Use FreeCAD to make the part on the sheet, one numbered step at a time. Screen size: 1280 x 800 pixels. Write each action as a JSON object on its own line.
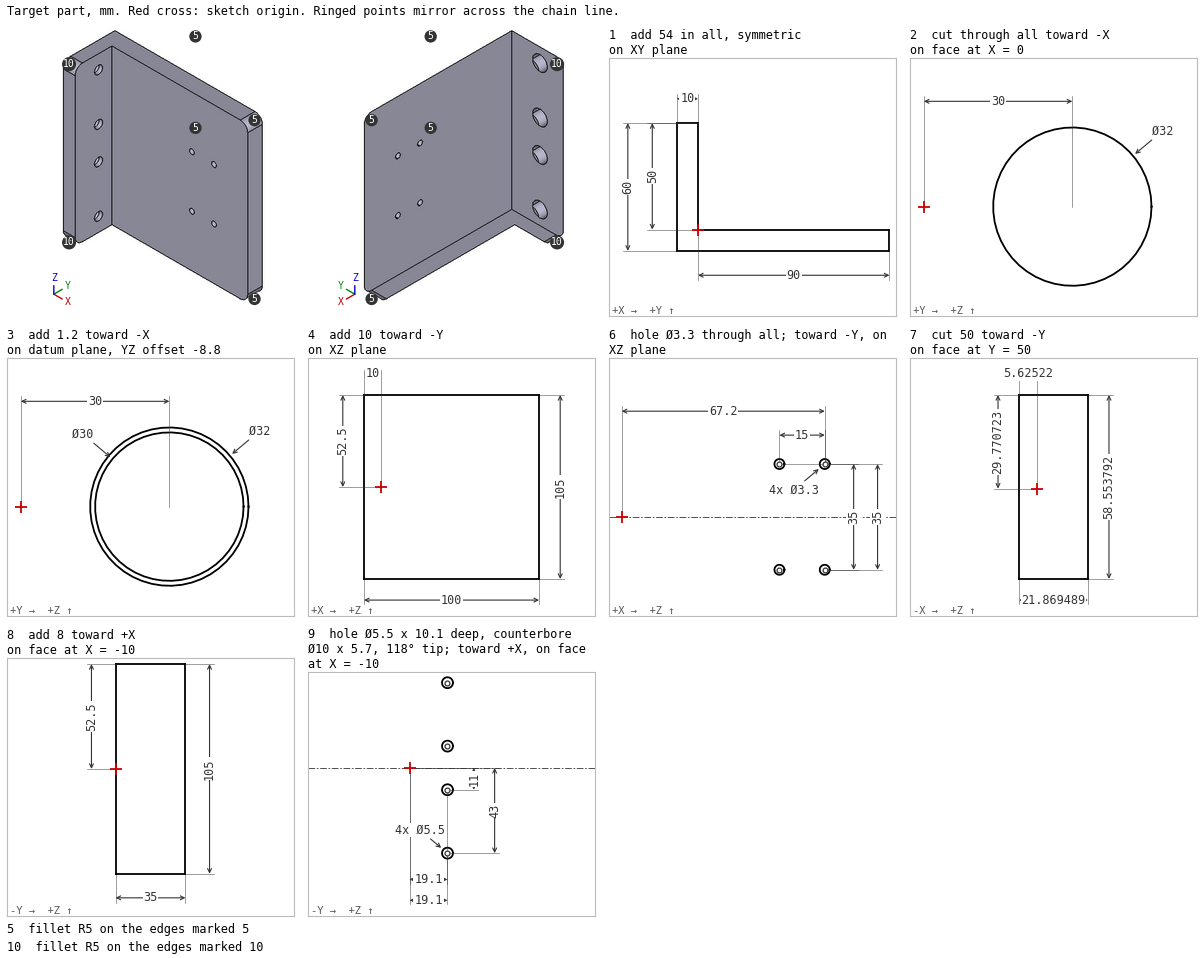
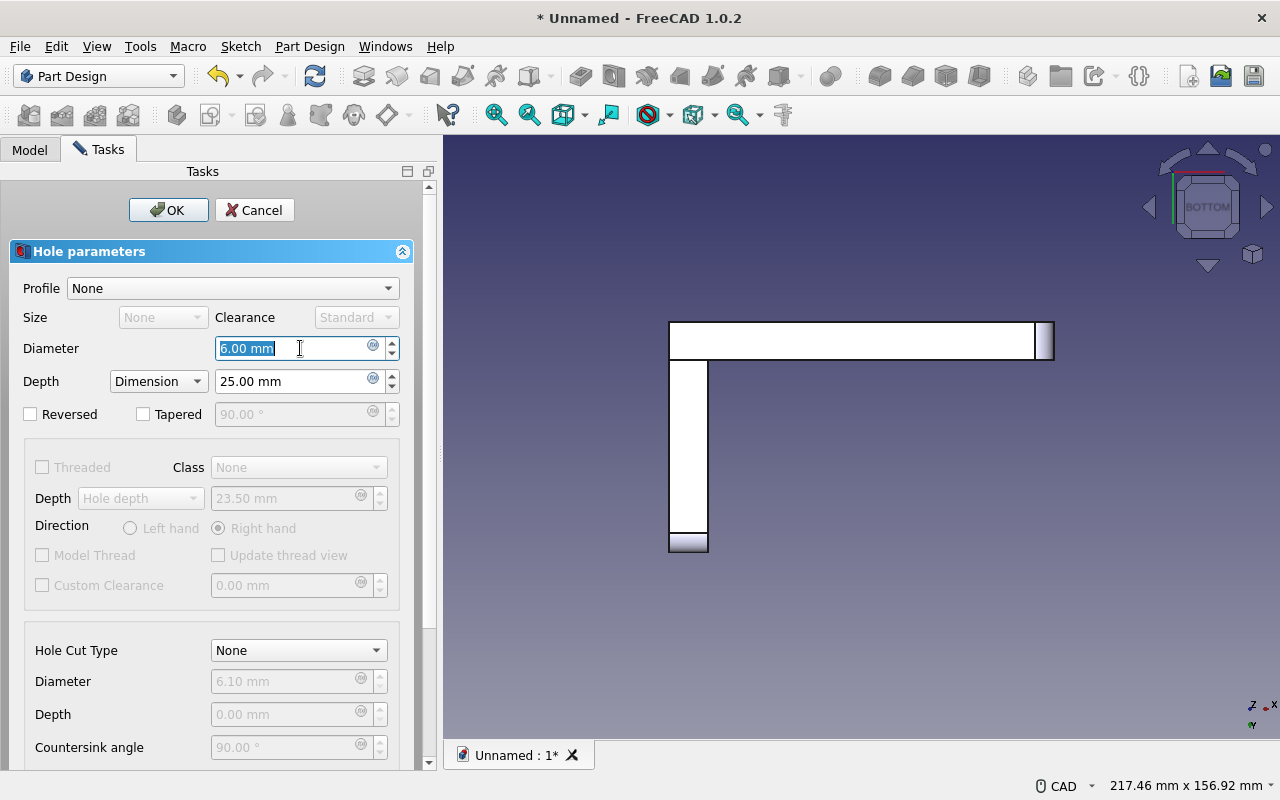
{"action": "type", "text": "3.3"}
{"action": "key", "text": "Tab"}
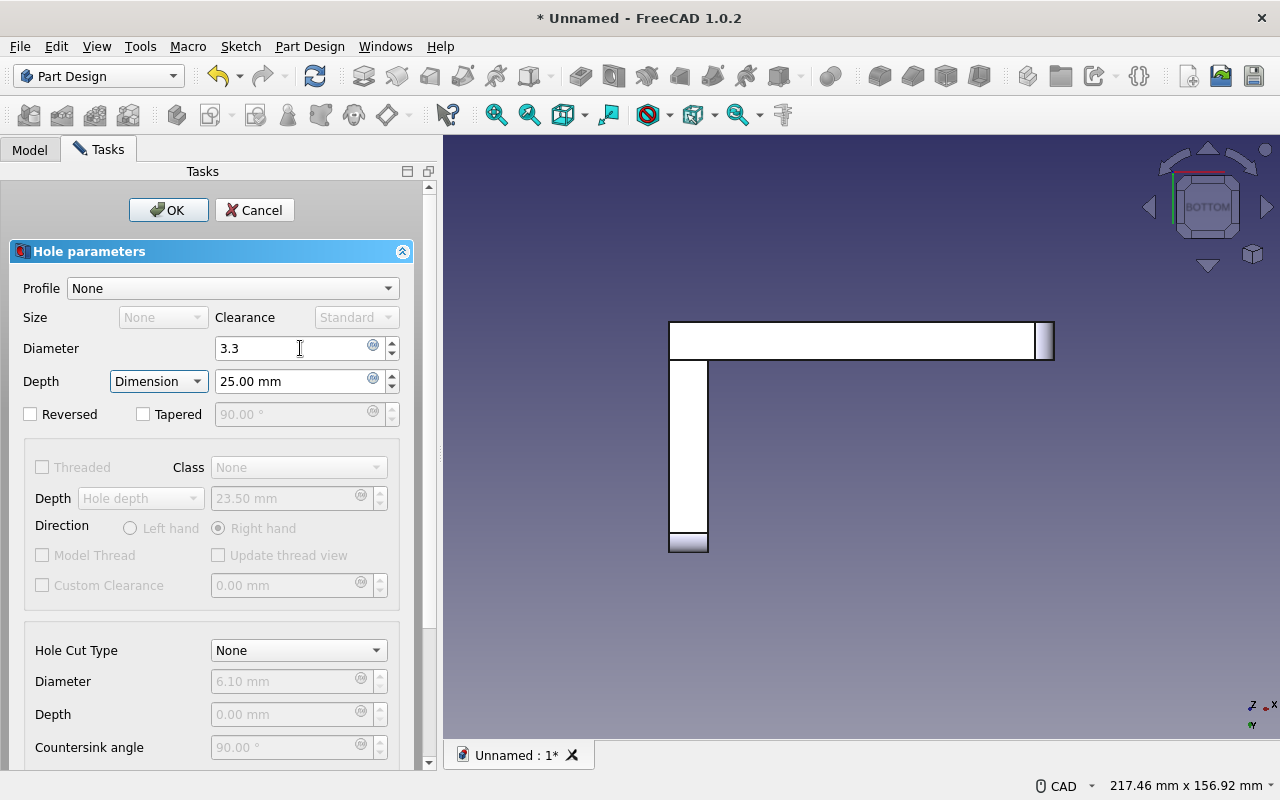
{"action": "left_click", "coordinate": [160, 382]}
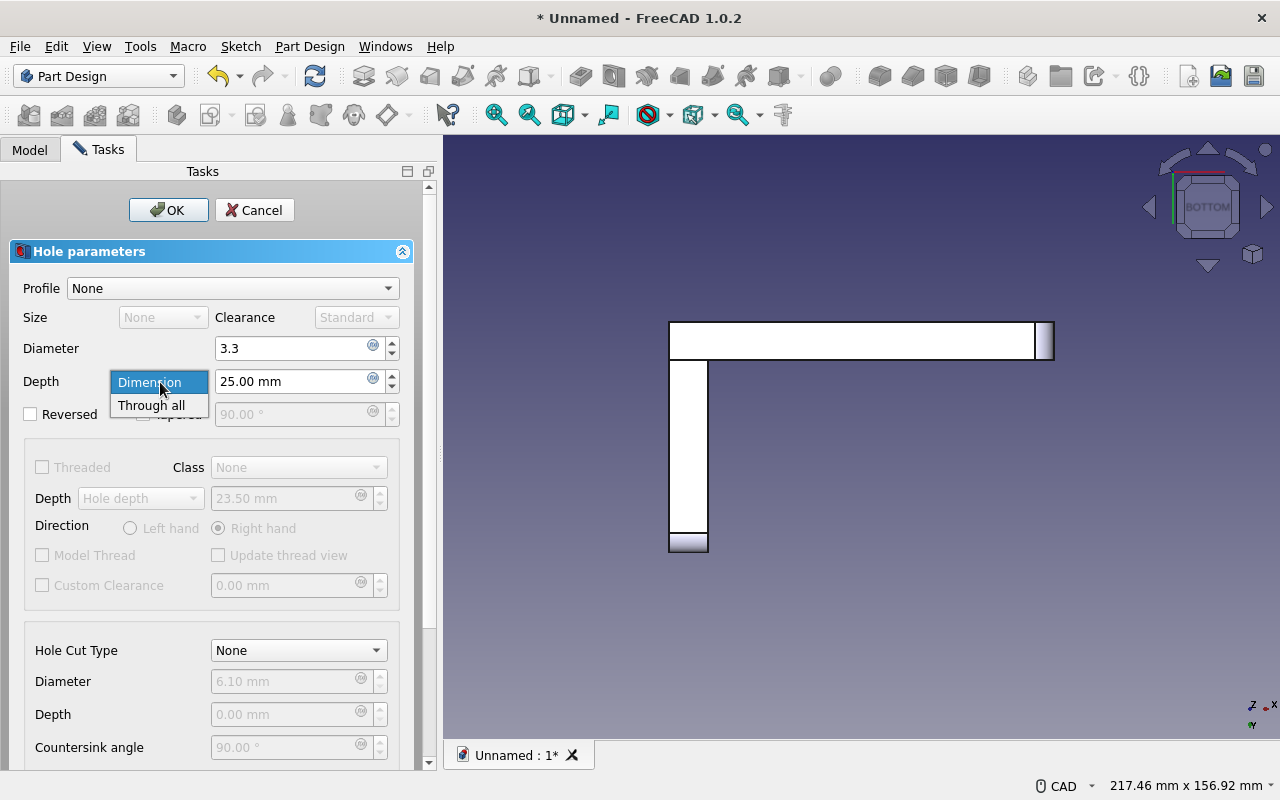
{"action": "left_click", "coordinate": [158, 406]}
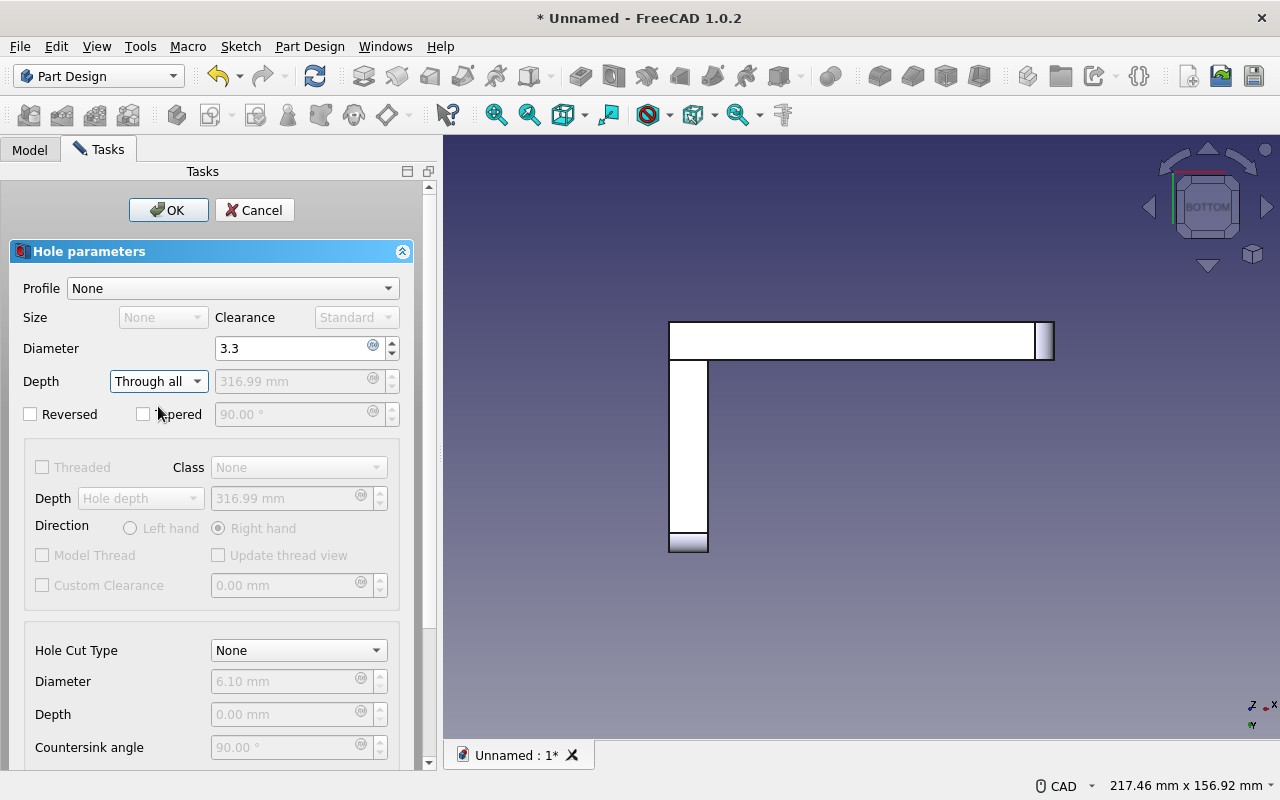
{"action": "left_click", "coordinate": [31, 414]}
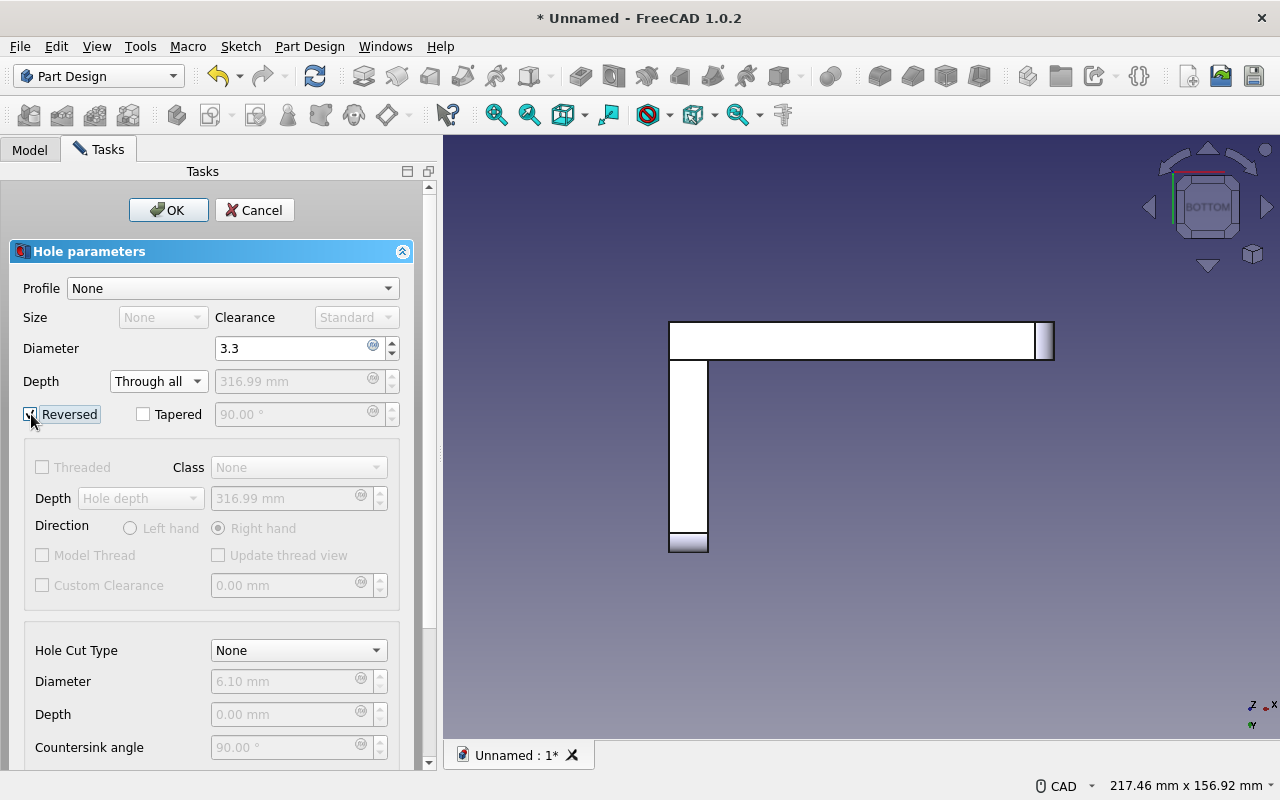
{"action": "left_click", "coordinate": [169, 210]}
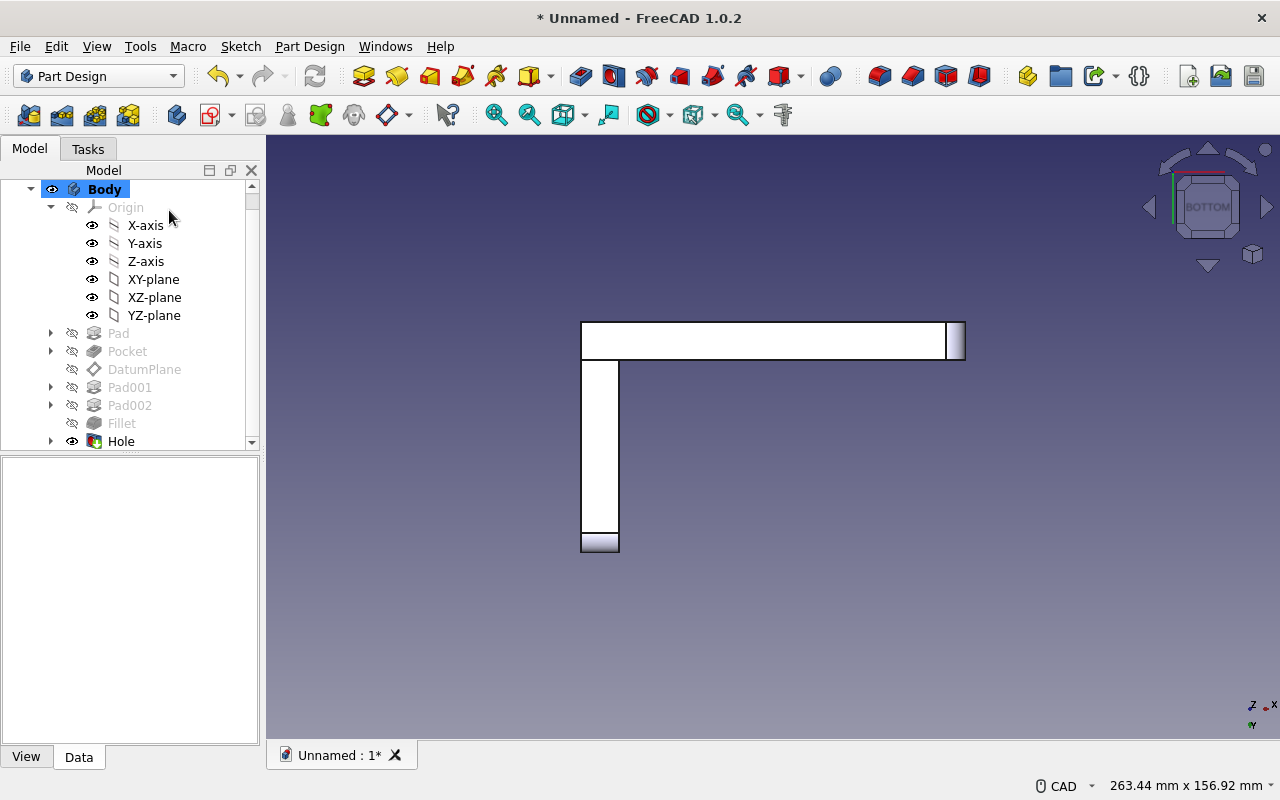
{"action": "left_click", "coordinate": [497, 116]}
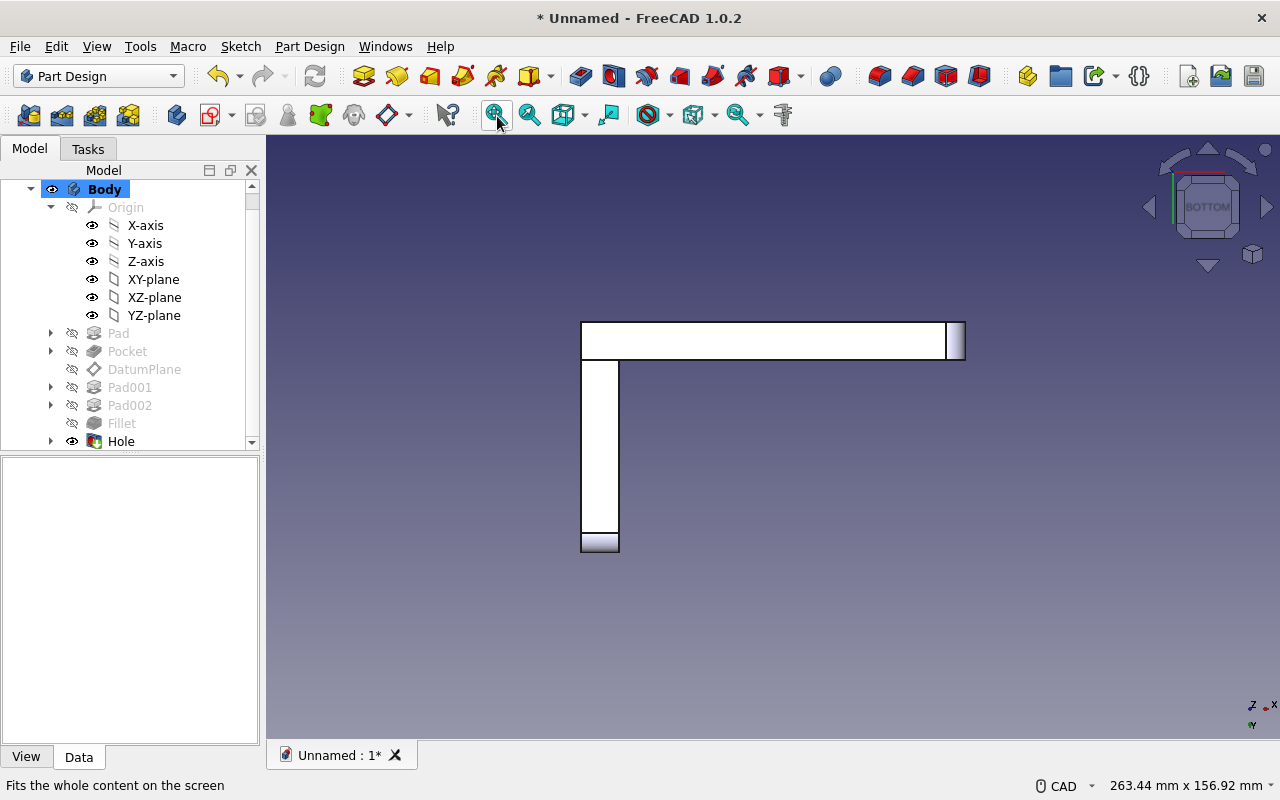
{"action": "key", "text": "4"}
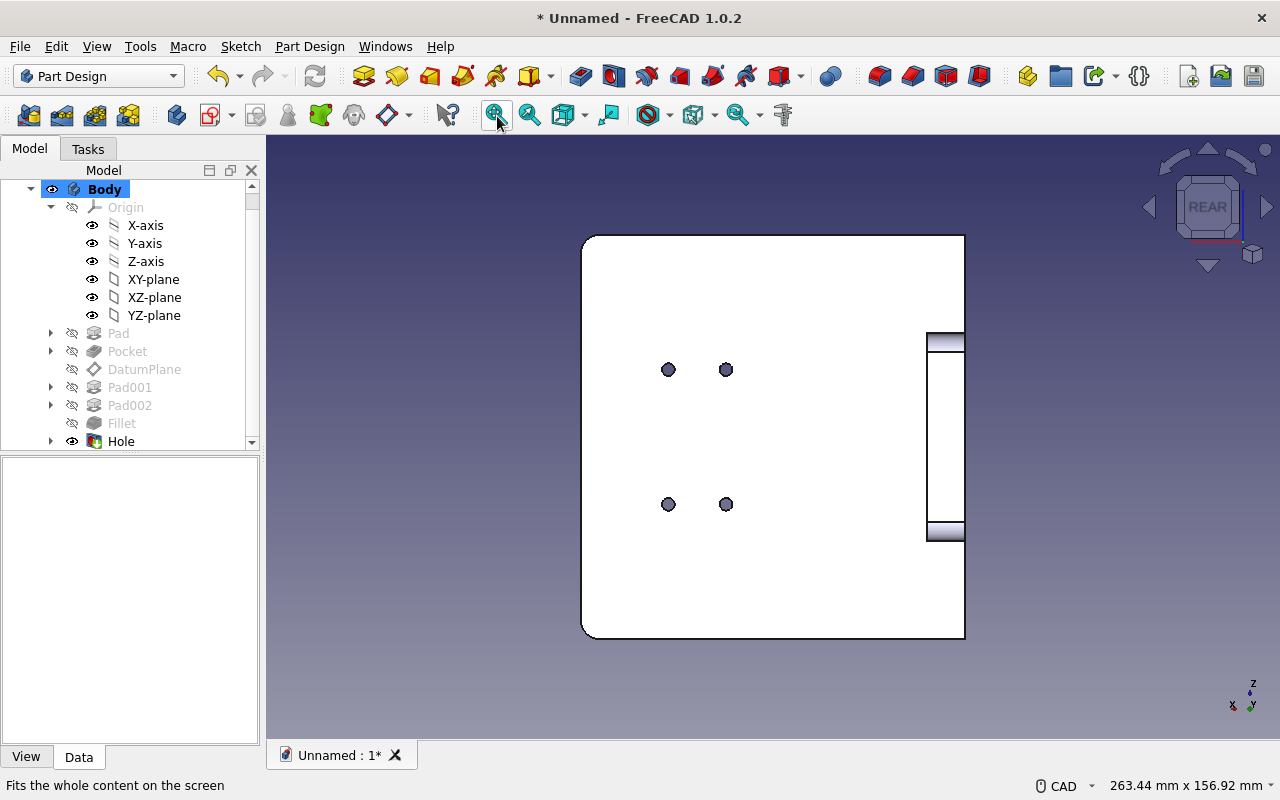
{"action": "left_click", "coordinate": [946, 388]}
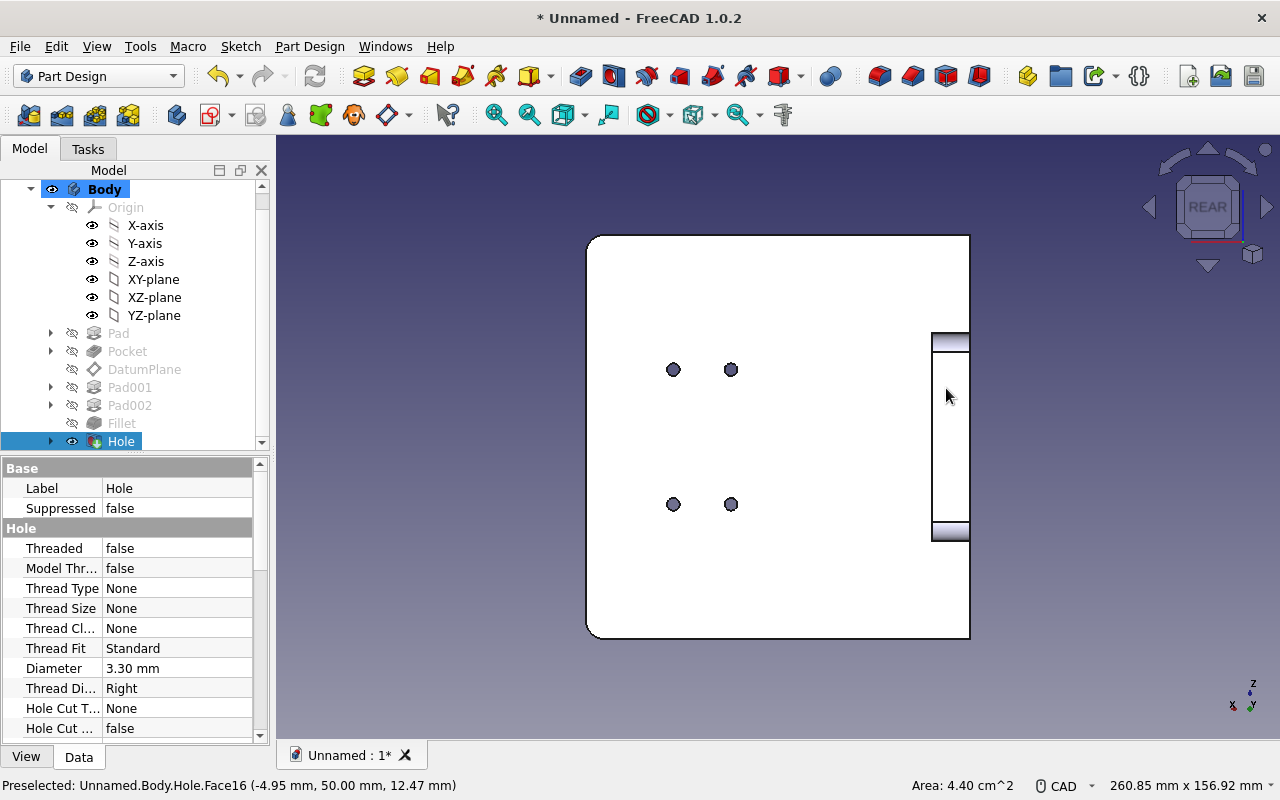
{"action": "left_click", "coordinate": [210, 116]}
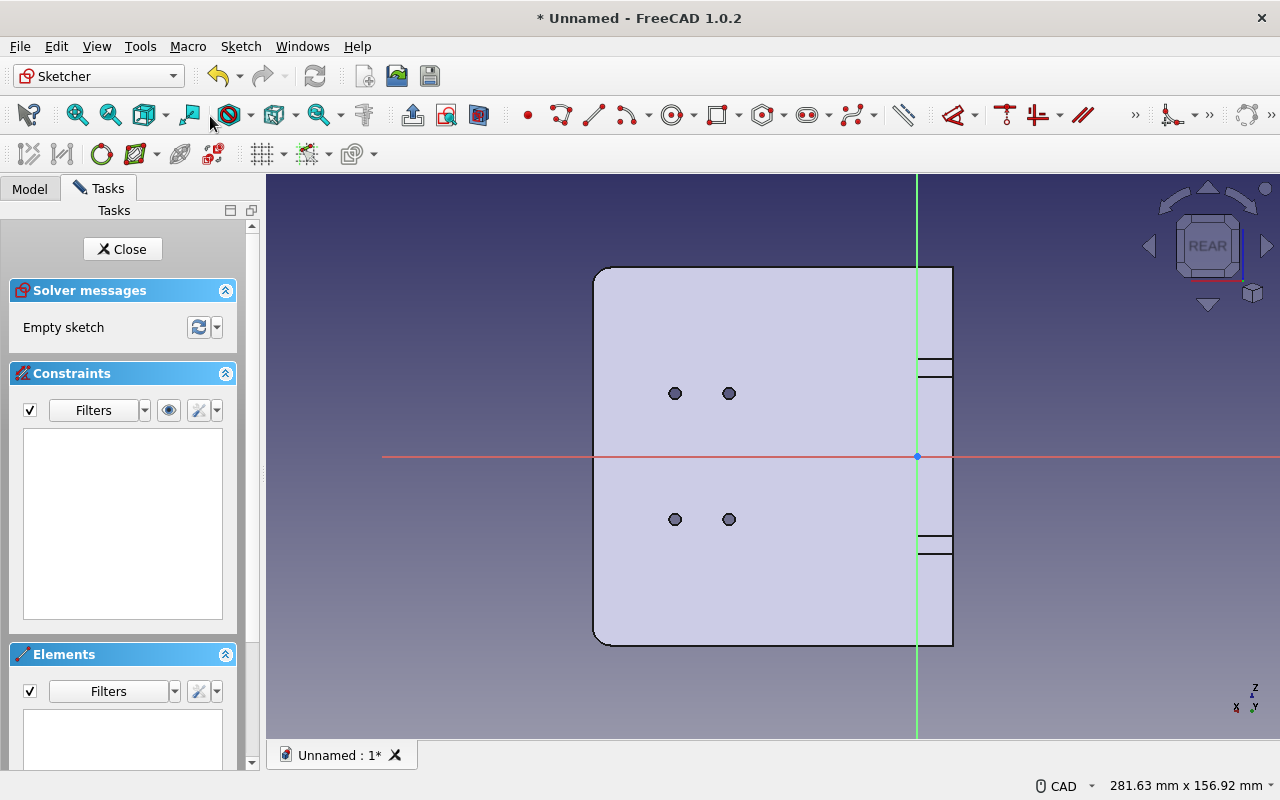
{"action": "scroll", "coordinate": [1115, 453], "scroll_direction": "up", "scroll_amount": 3}